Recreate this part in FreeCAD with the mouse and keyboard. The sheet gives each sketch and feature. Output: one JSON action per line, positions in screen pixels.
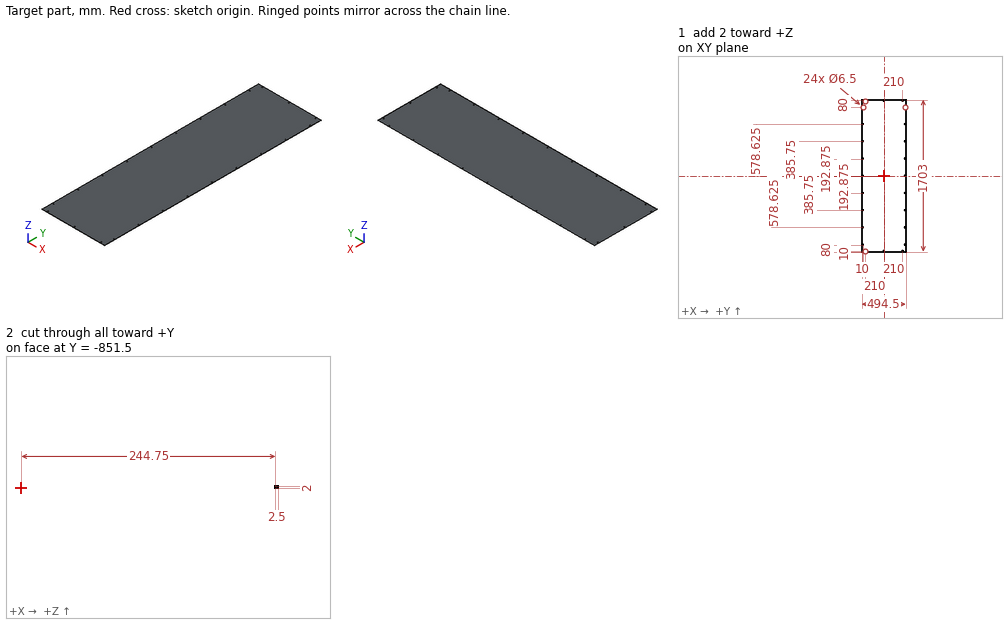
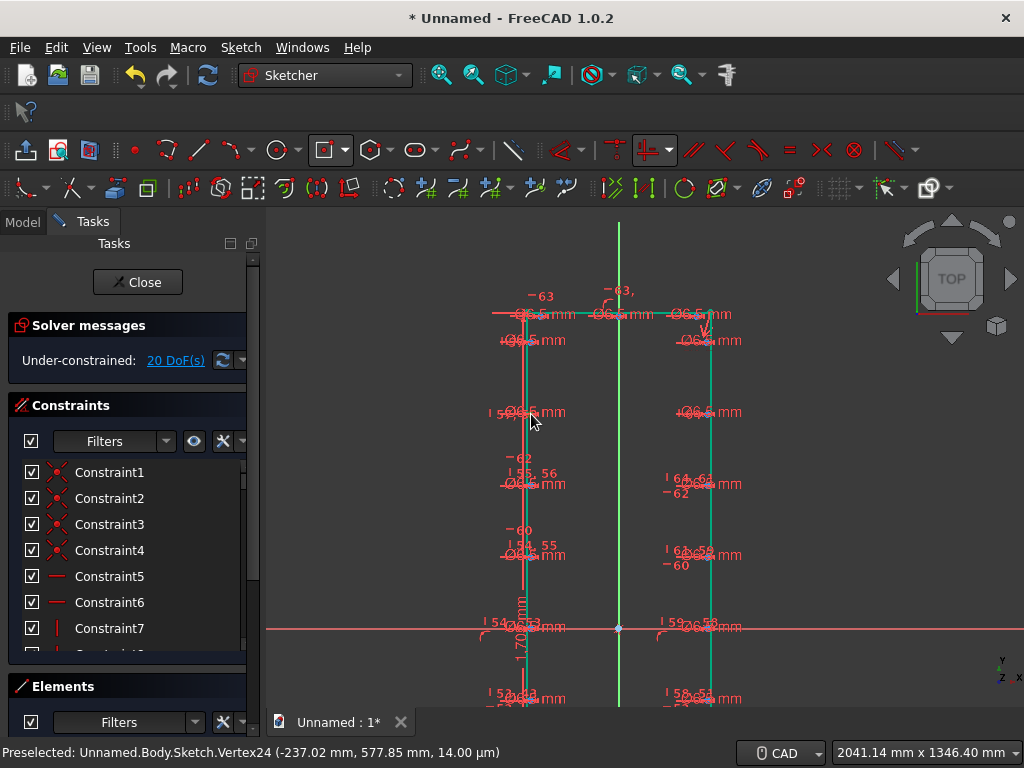
{"action": "left_click", "coordinate": [707, 414]}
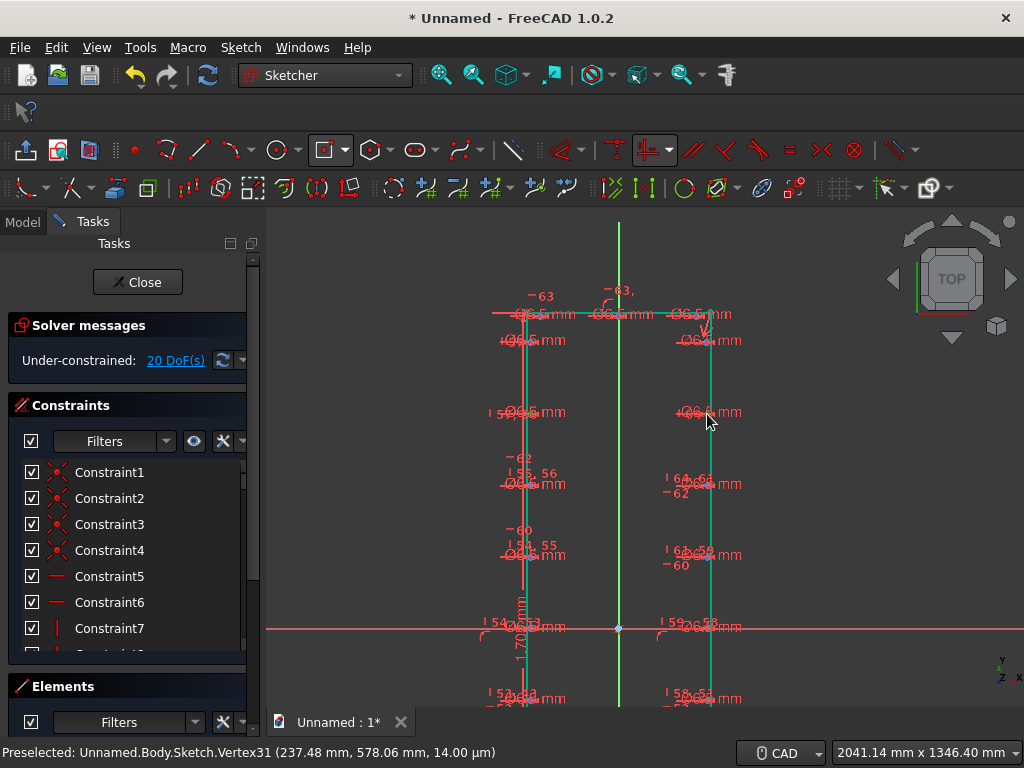
{"action": "key", "text": "h"}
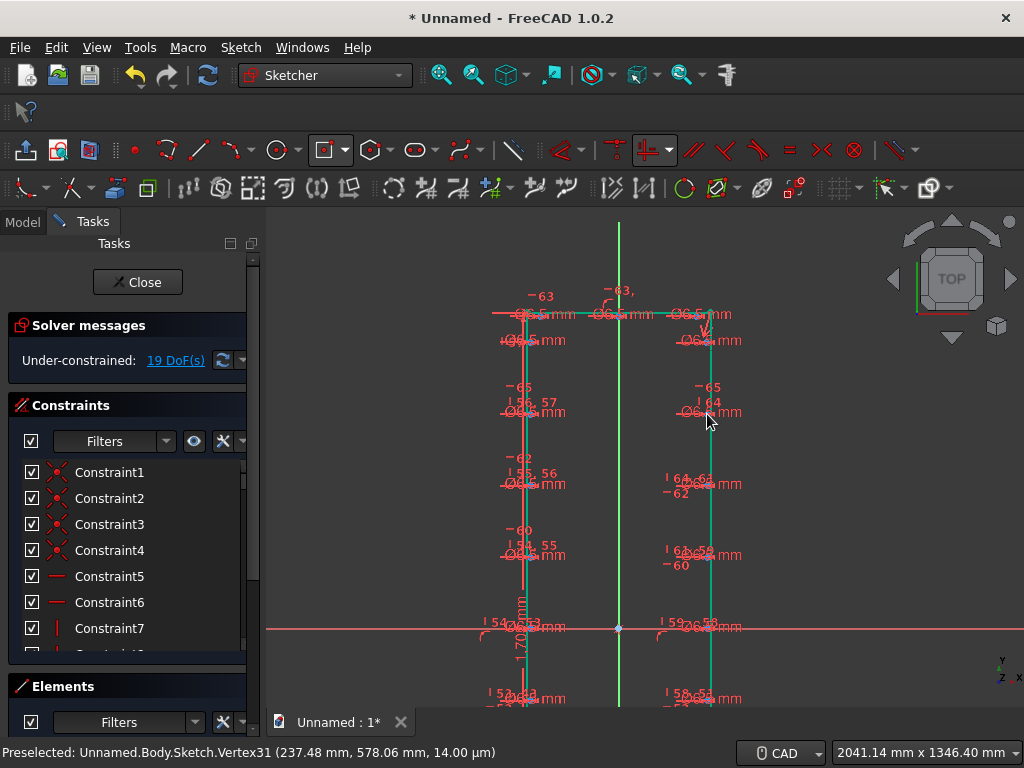
{"action": "left_click", "coordinate": [619, 316]}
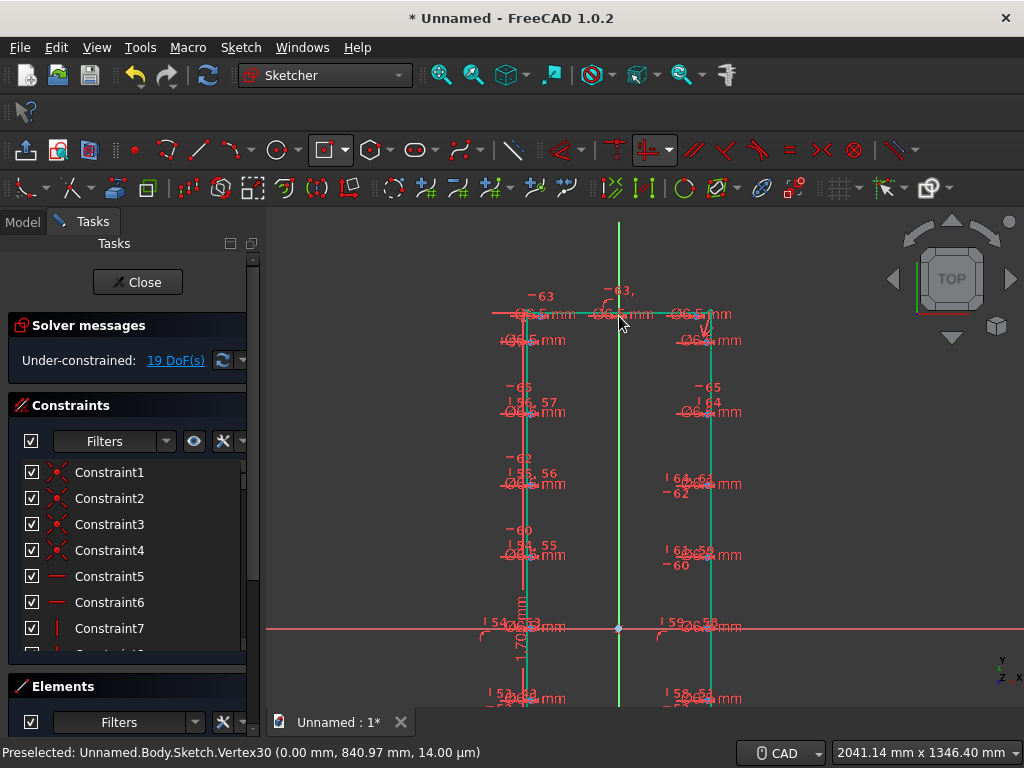
{"action": "left_click", "coordinate": [697, 316]}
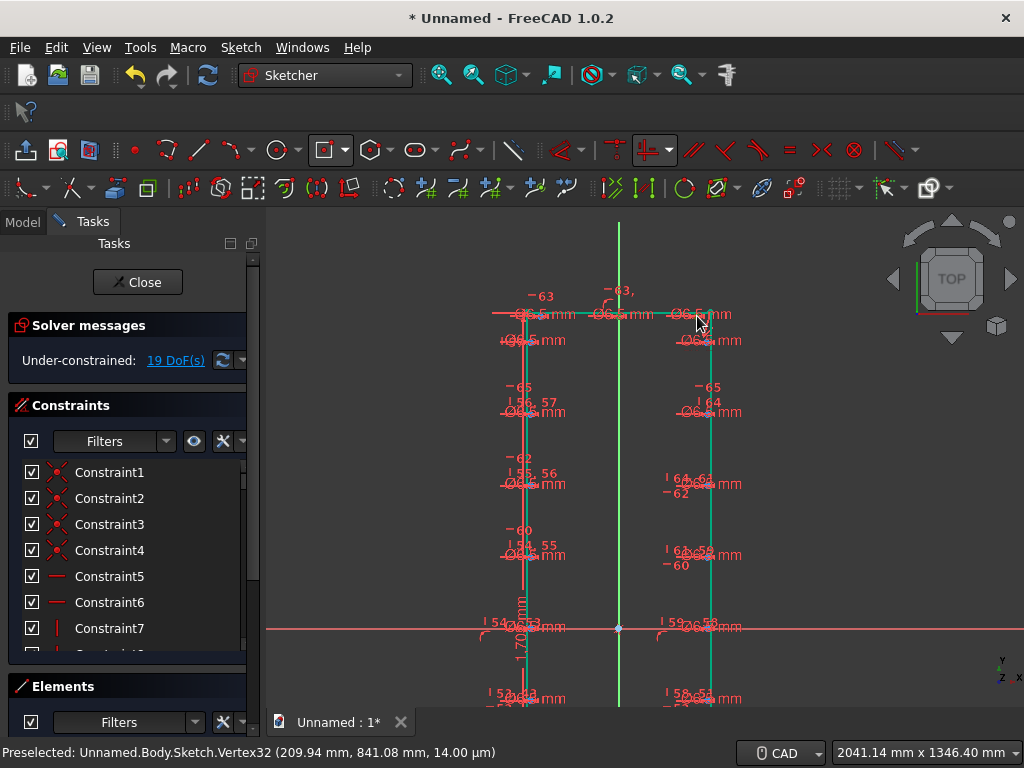
{"action": "left_click", "coordinate": [672, 150]}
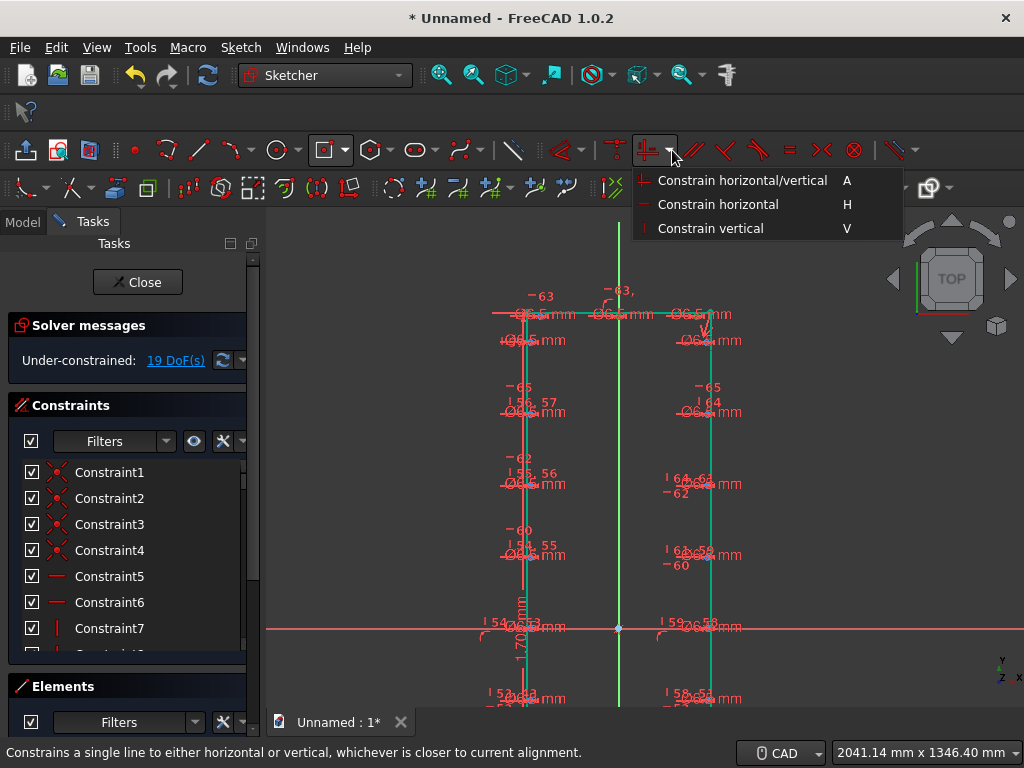
{"action": "left_click", "coordinate": [768, 204]}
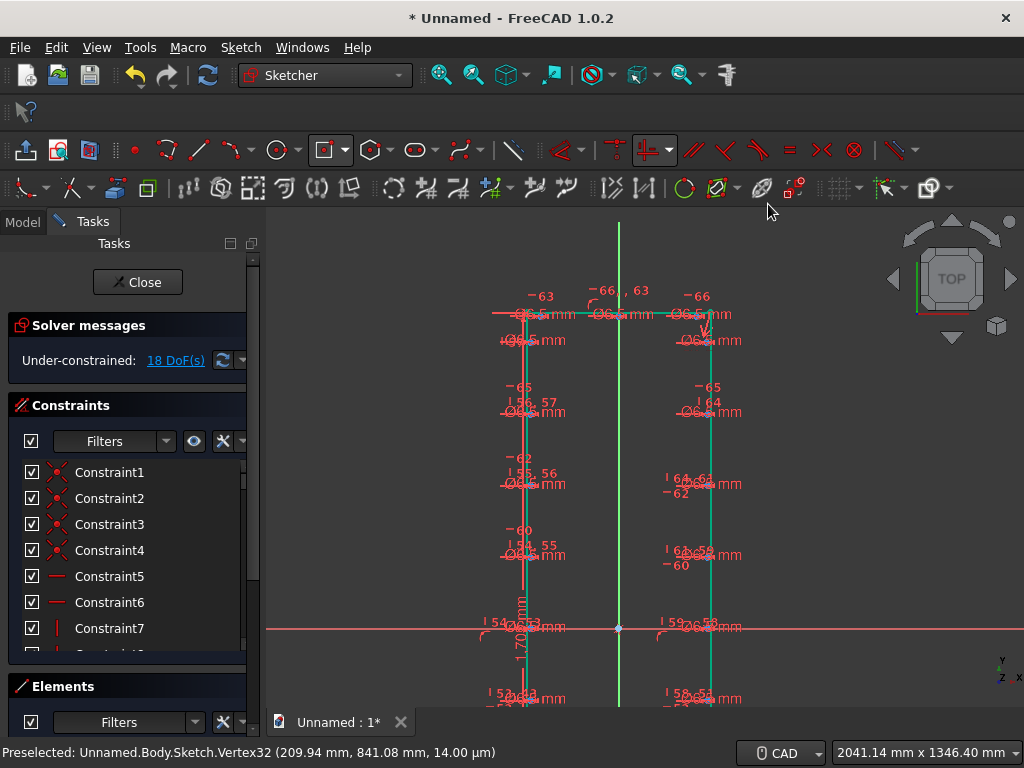
{"action": "left_click", "coordinate": [707, 414]}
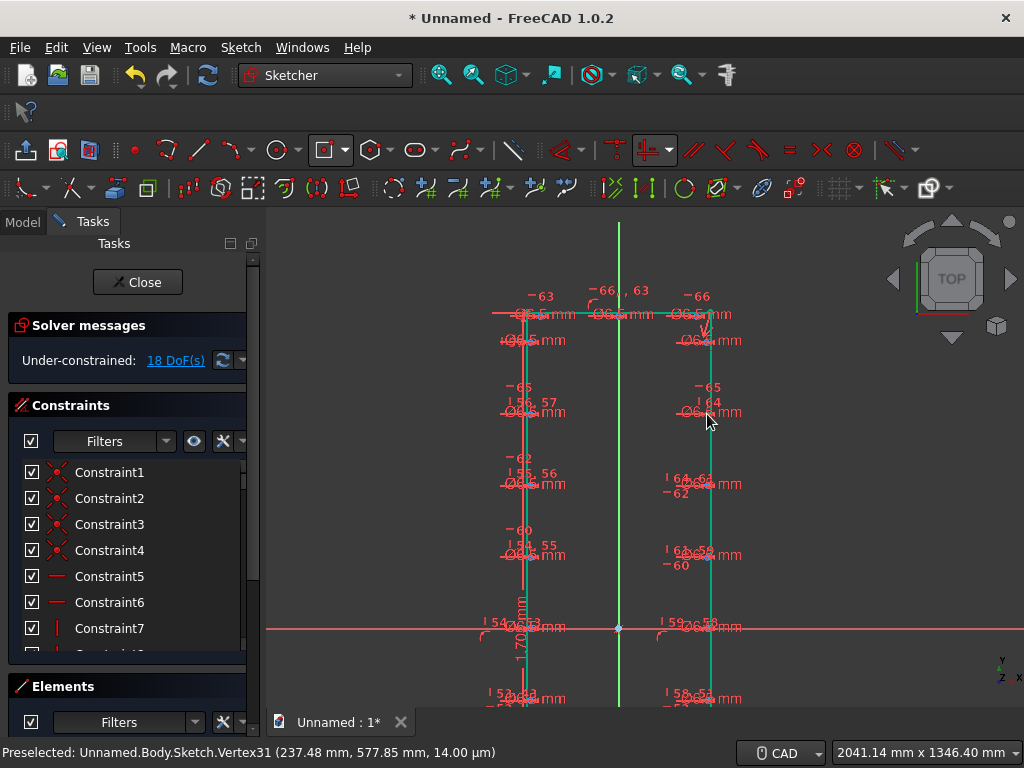
{"action": "left_click", "coordinate": [707, 343]}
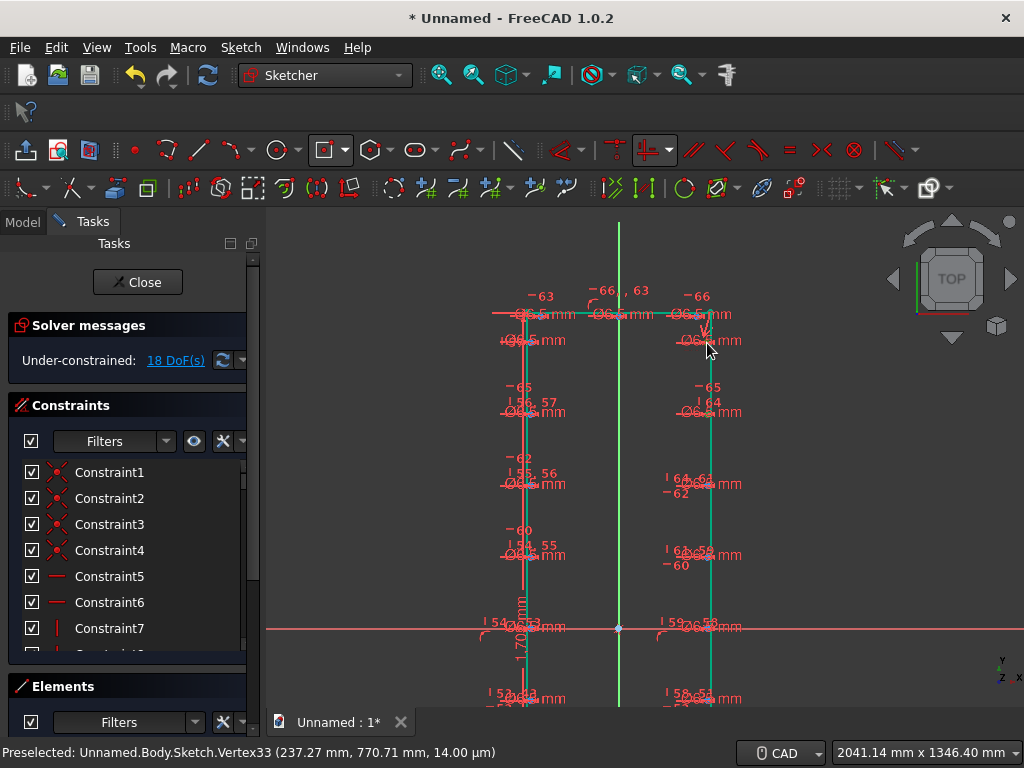
{"action": "left_click", "coordinate": [672, 150]}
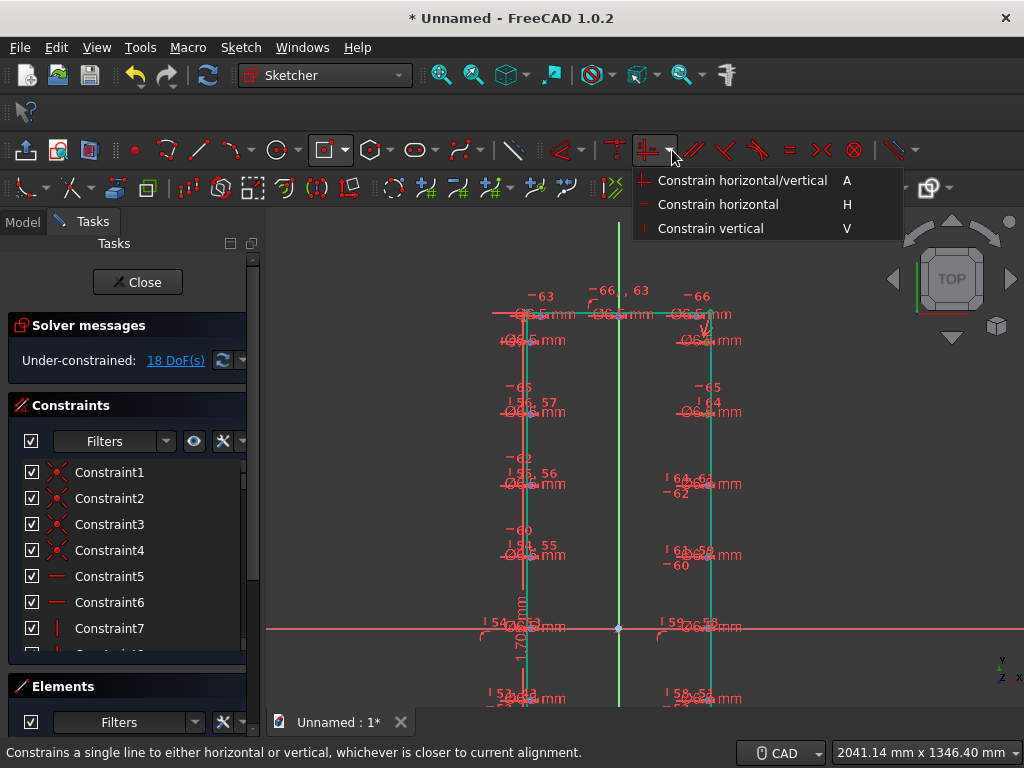
{"action": "left_click", "coordinate": [768, 228]}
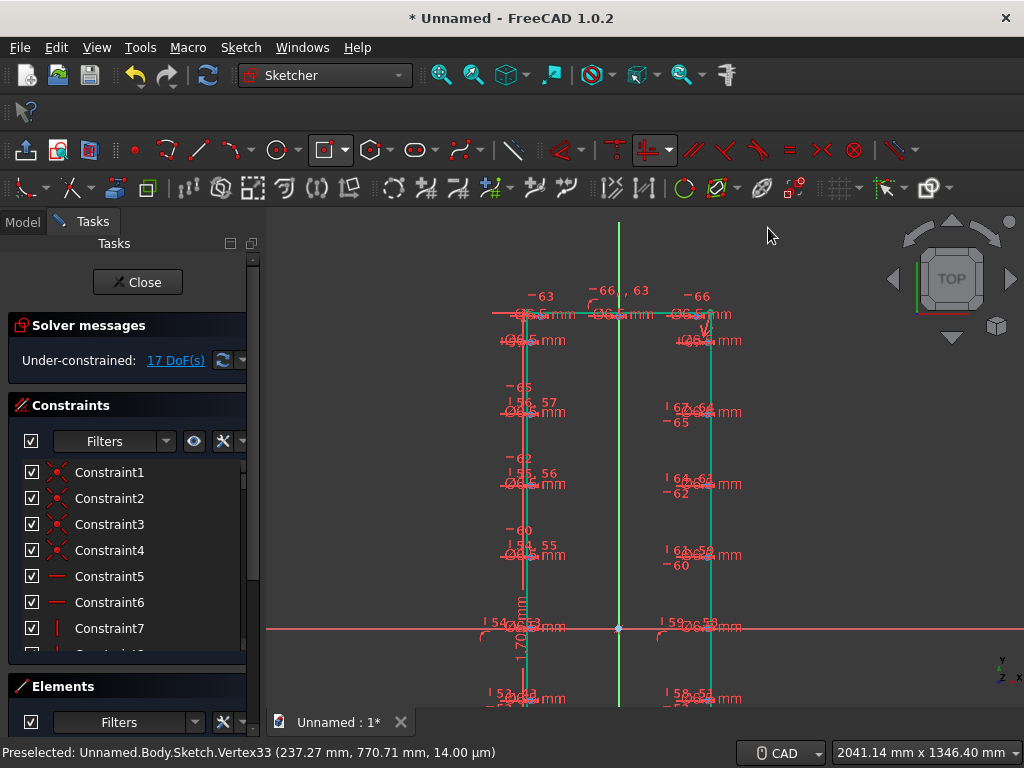
{"action": "scroll", "coordinate": [542, 317], "scroll_direction": "down", "scroll_amount": 4}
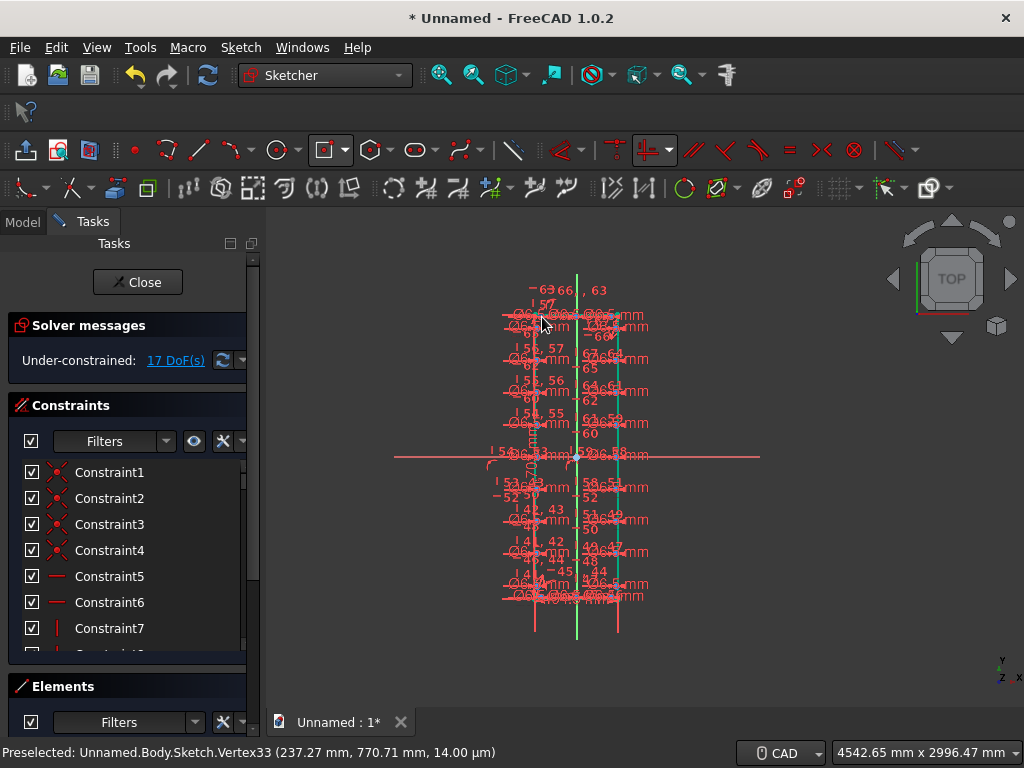
{"action": "scroll", "coordinate": [542, 598], "scroll_direction": "up", "scroll_amount": 4}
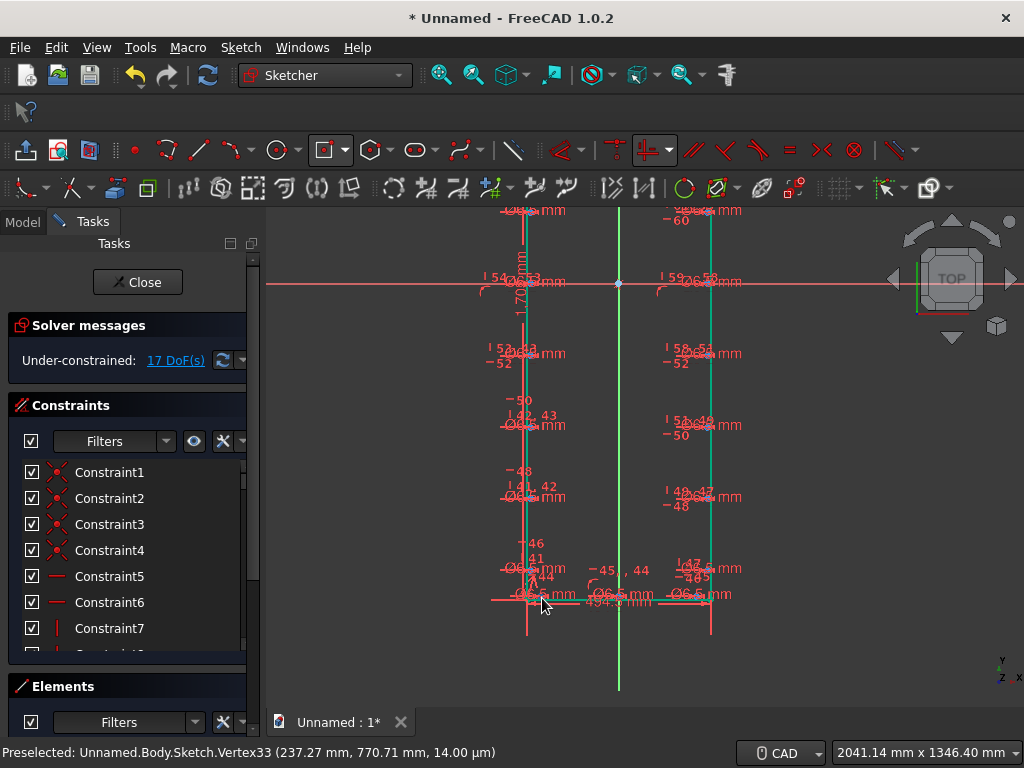
{"action": "left_click", "coordinate": [541, 596]}